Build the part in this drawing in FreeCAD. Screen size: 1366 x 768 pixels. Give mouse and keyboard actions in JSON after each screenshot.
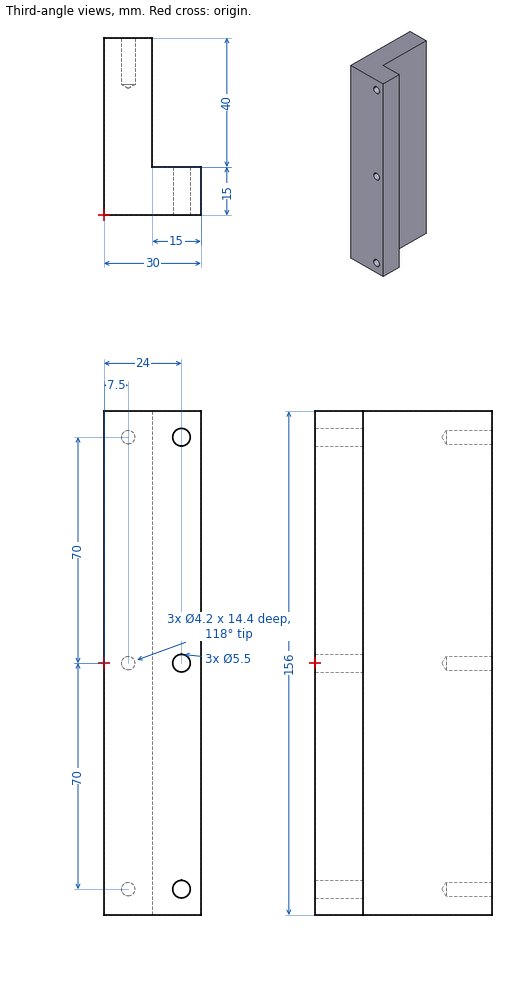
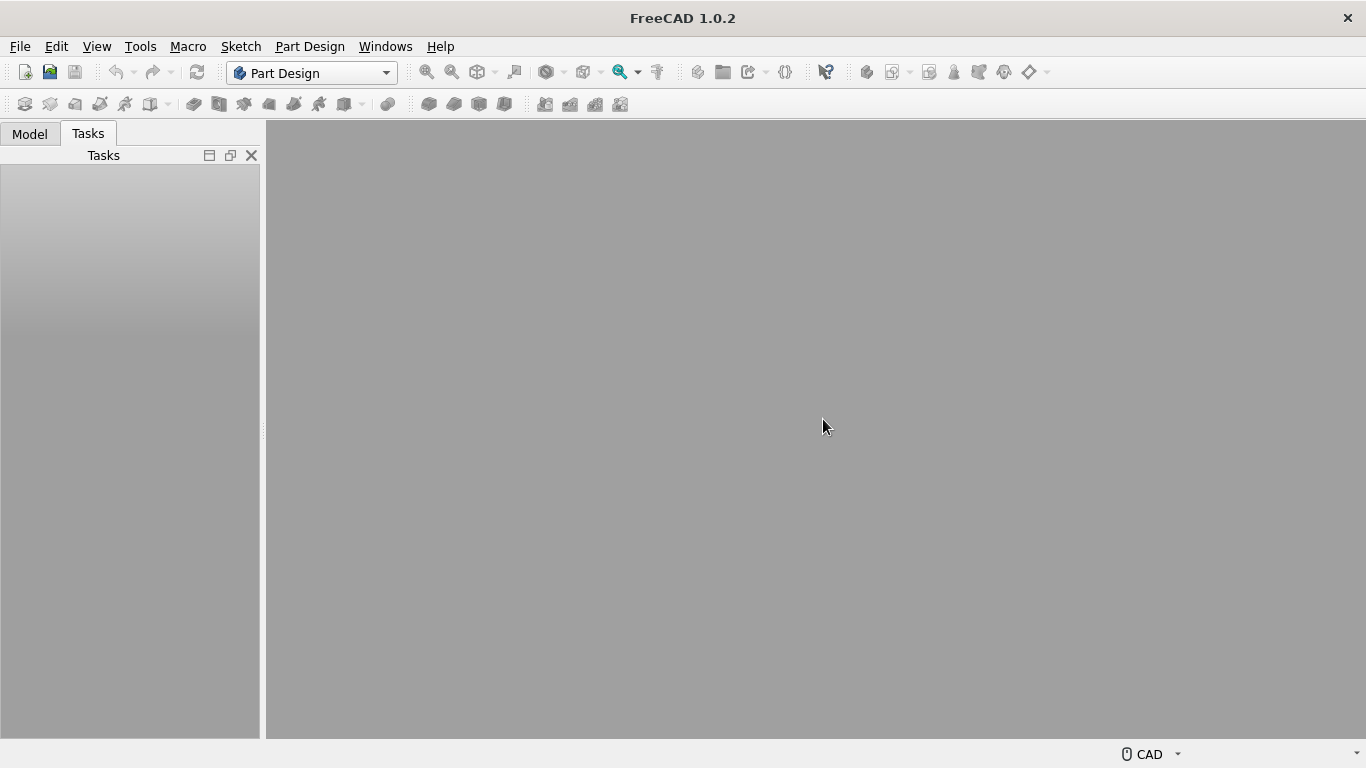
{"action": "key", "text": "ctrl+n"}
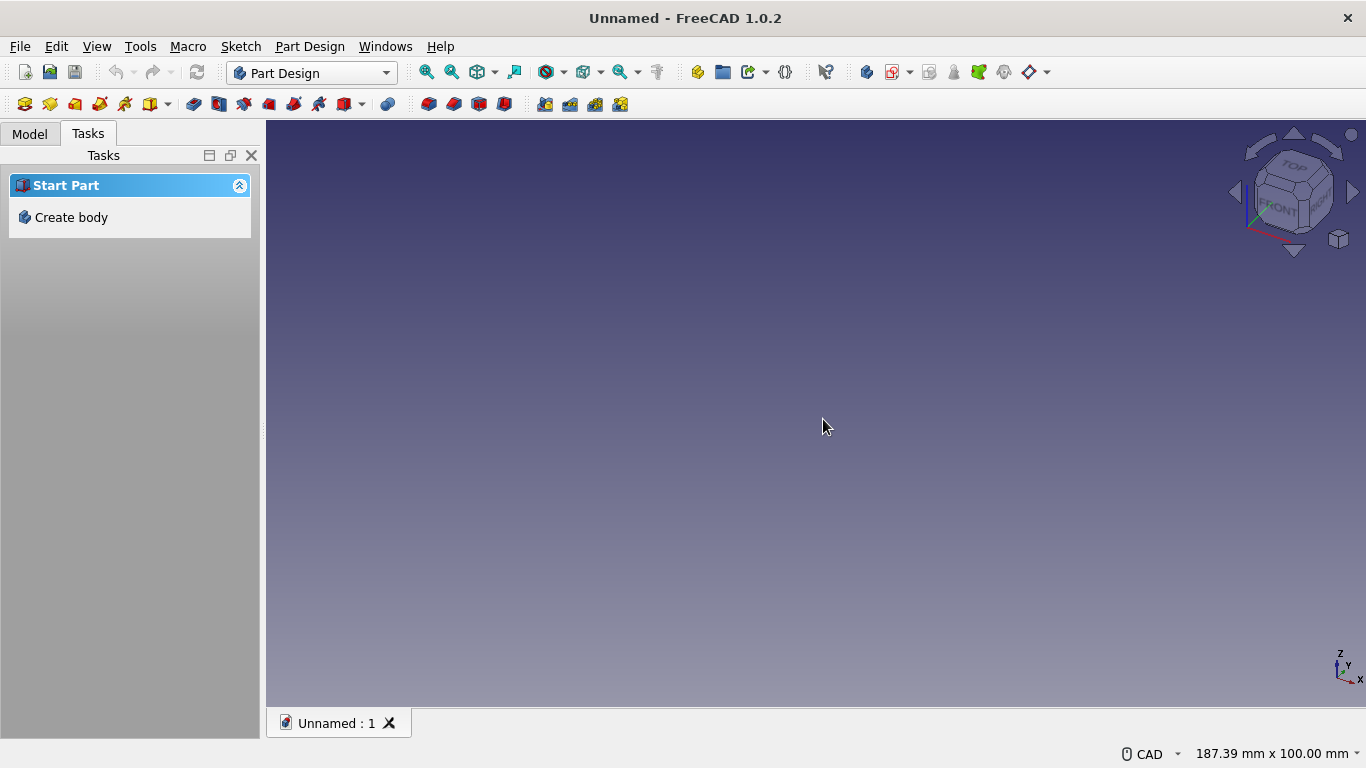
{"action": "left_click", "coordinate": [892, 72]}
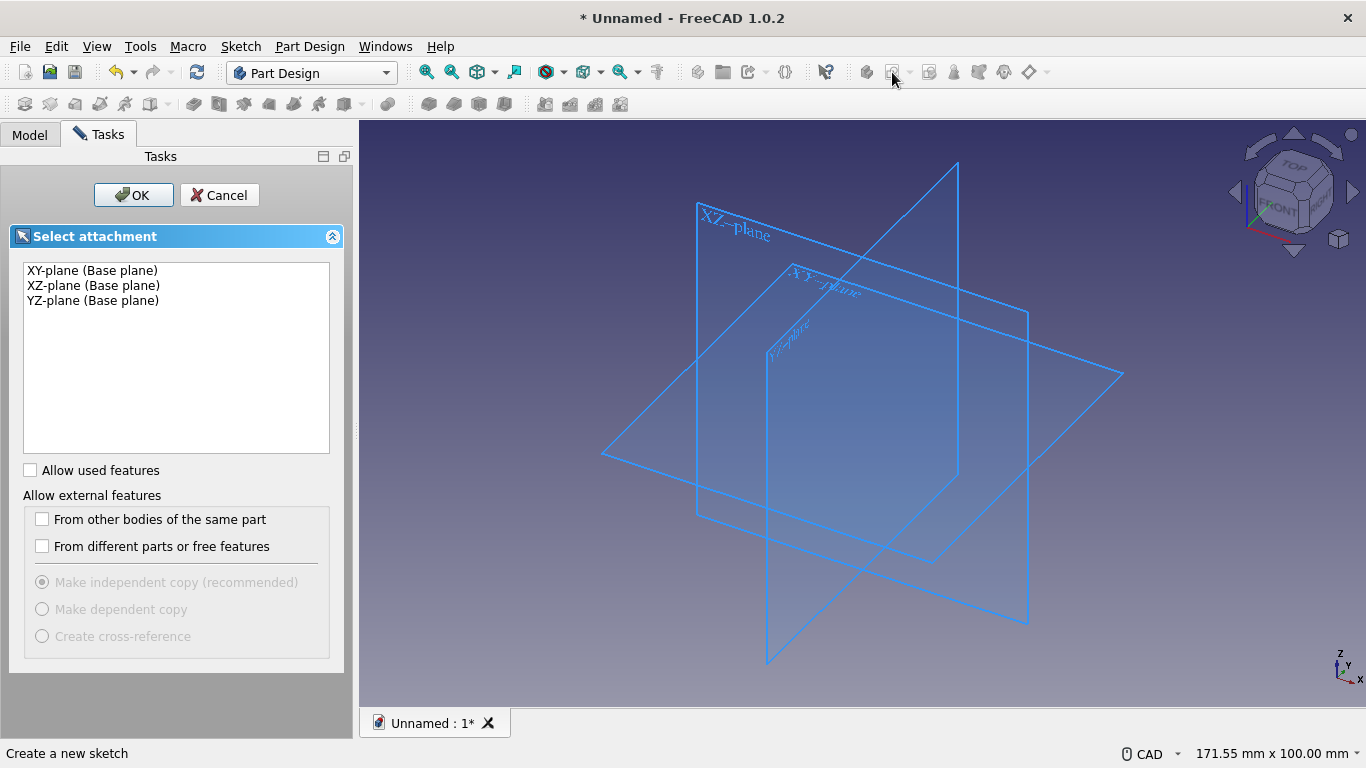
{"action": "left_click", "coordinate": [84, 270]}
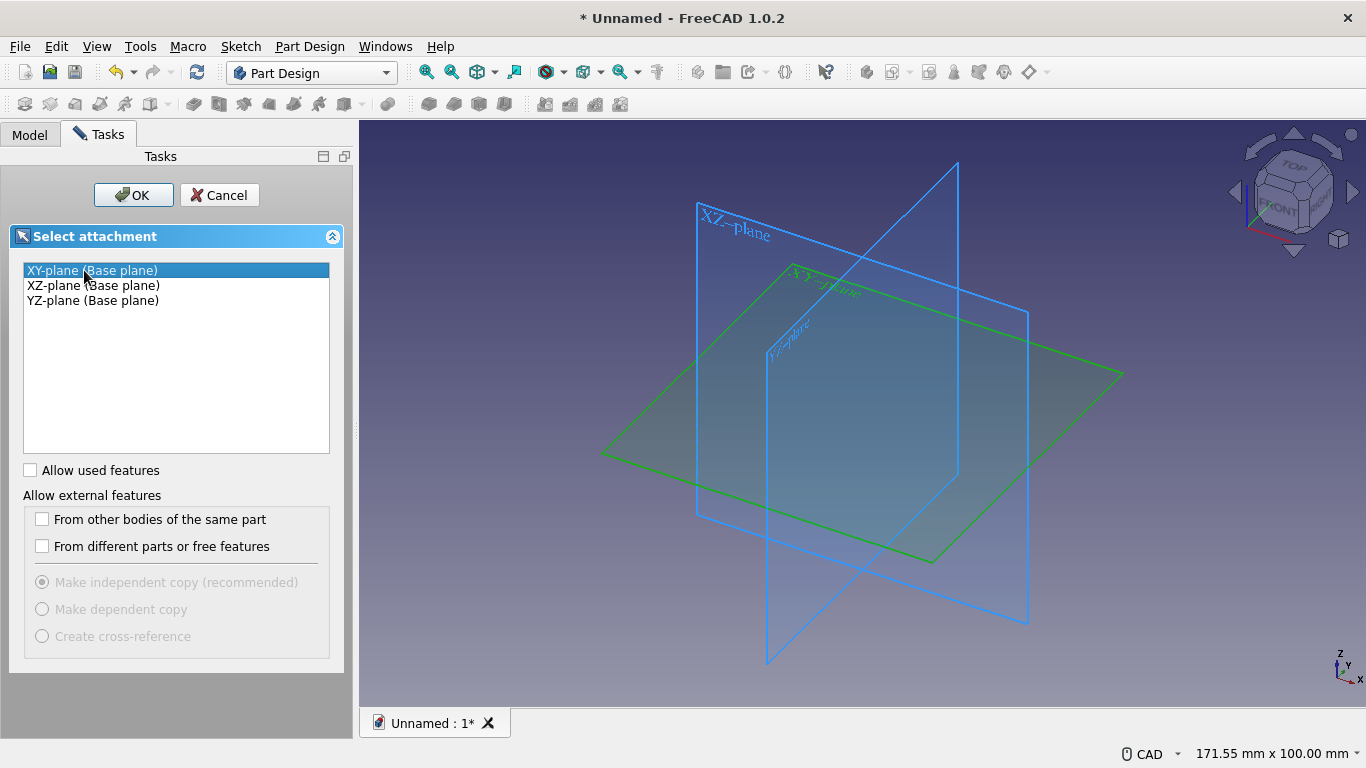
{"action": "left_click", "coordinate": [134, 195]}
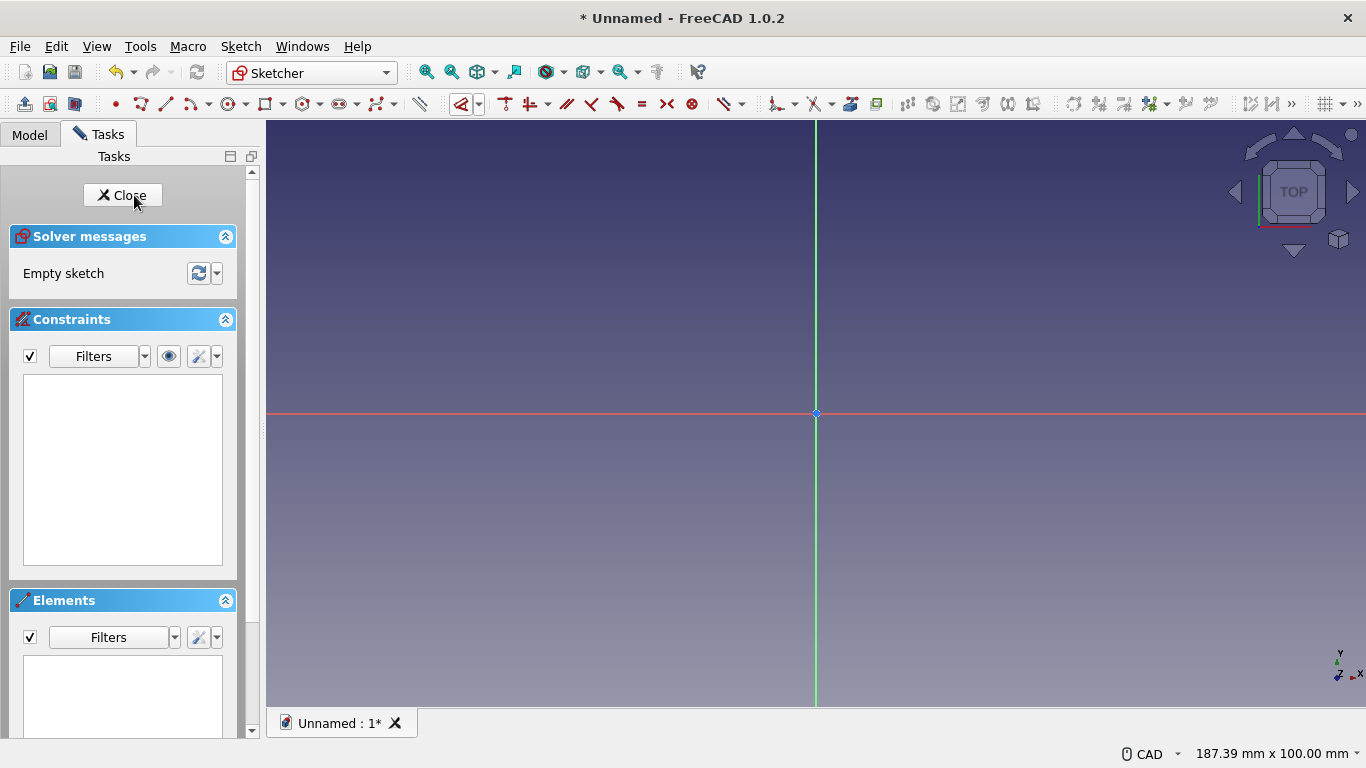
{"action": "scroll", "coordinate": [294, 679], "scroll_direction": "down", "scroll_amount": 1}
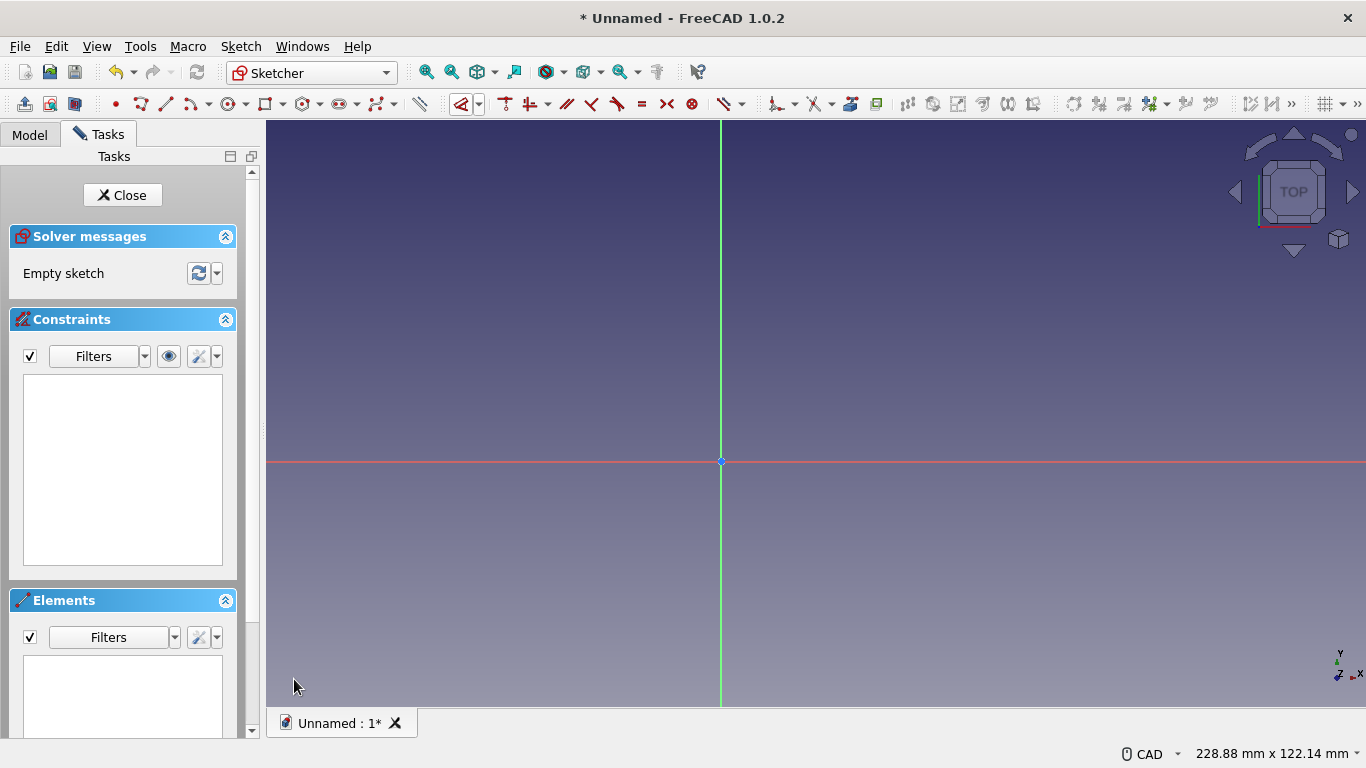
{"action": "scroll", "coordinate": [887, 159], "scroll_direction": "up", "scroll_amount": 2}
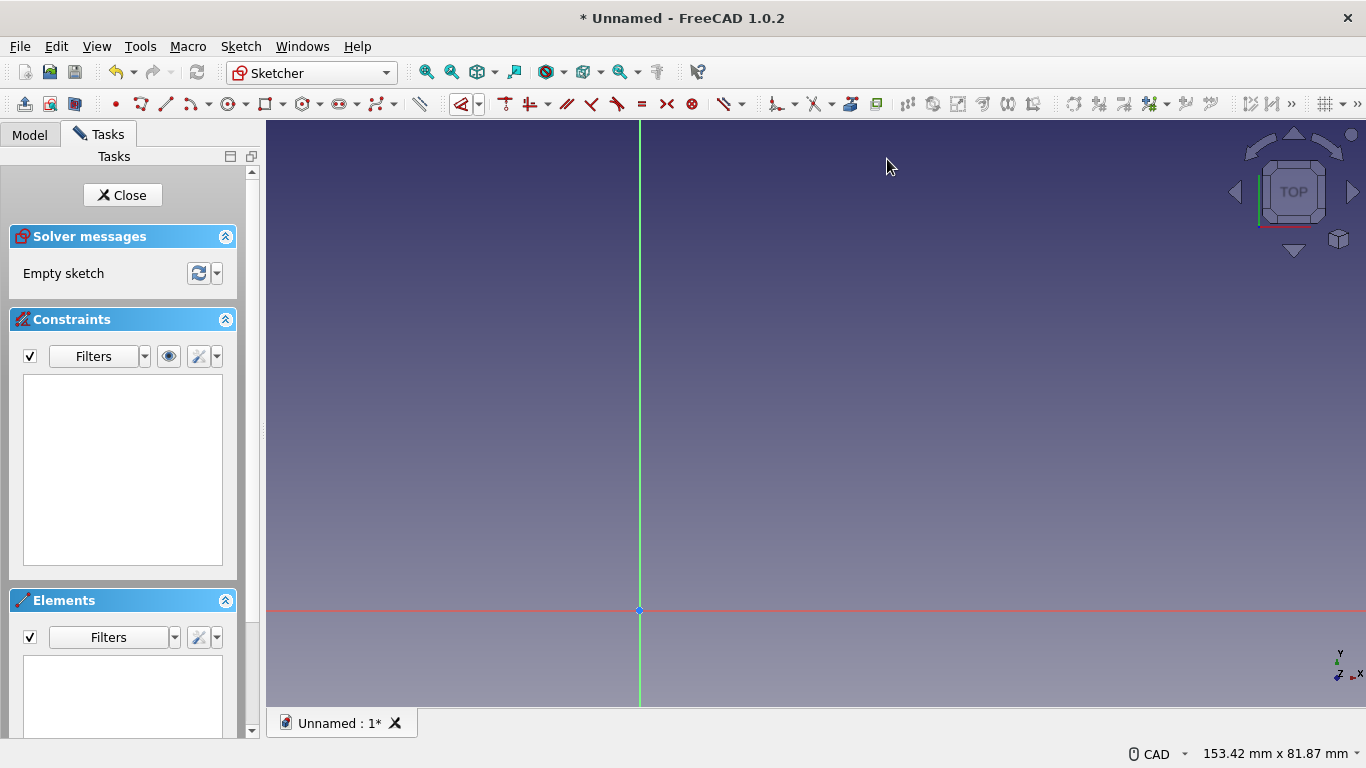
{"action": "key", "text": "g m"}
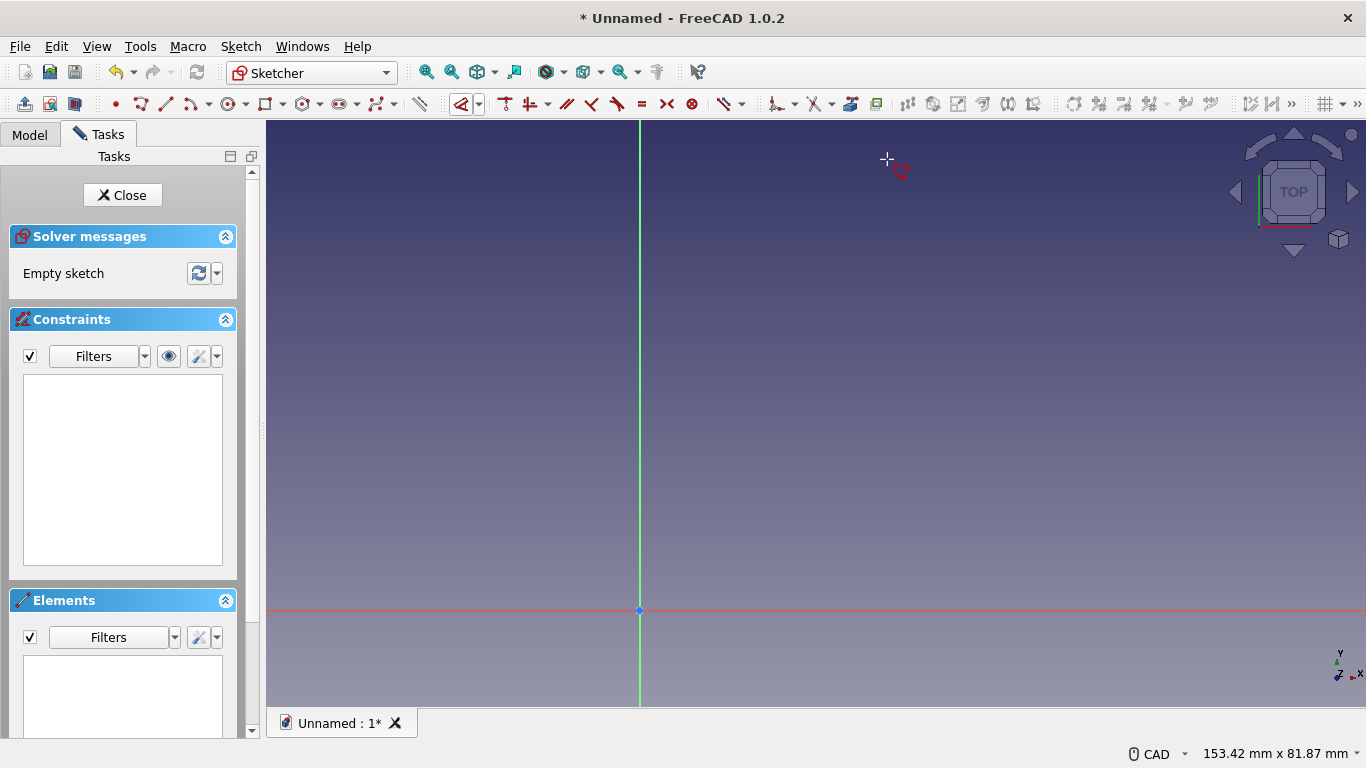
{"action": "left_click", "coordinate": [640, 611]}
{"action": "left_click", "coordinate": [855, 602]}
{"action": "left_click", "coordinate": [855, 503]}
{"action": "left_click", "coordinate": [747, 503]}
{"action": "left_click", "coordinate": [747, 216]}
{"action": "left_click", "coordinate": [649, 216]}
{"action": "left_click", "coordinate": [640, 611]}
{"action": "key", "text": "Escape"}
{"action": "key", "text": "Escape"}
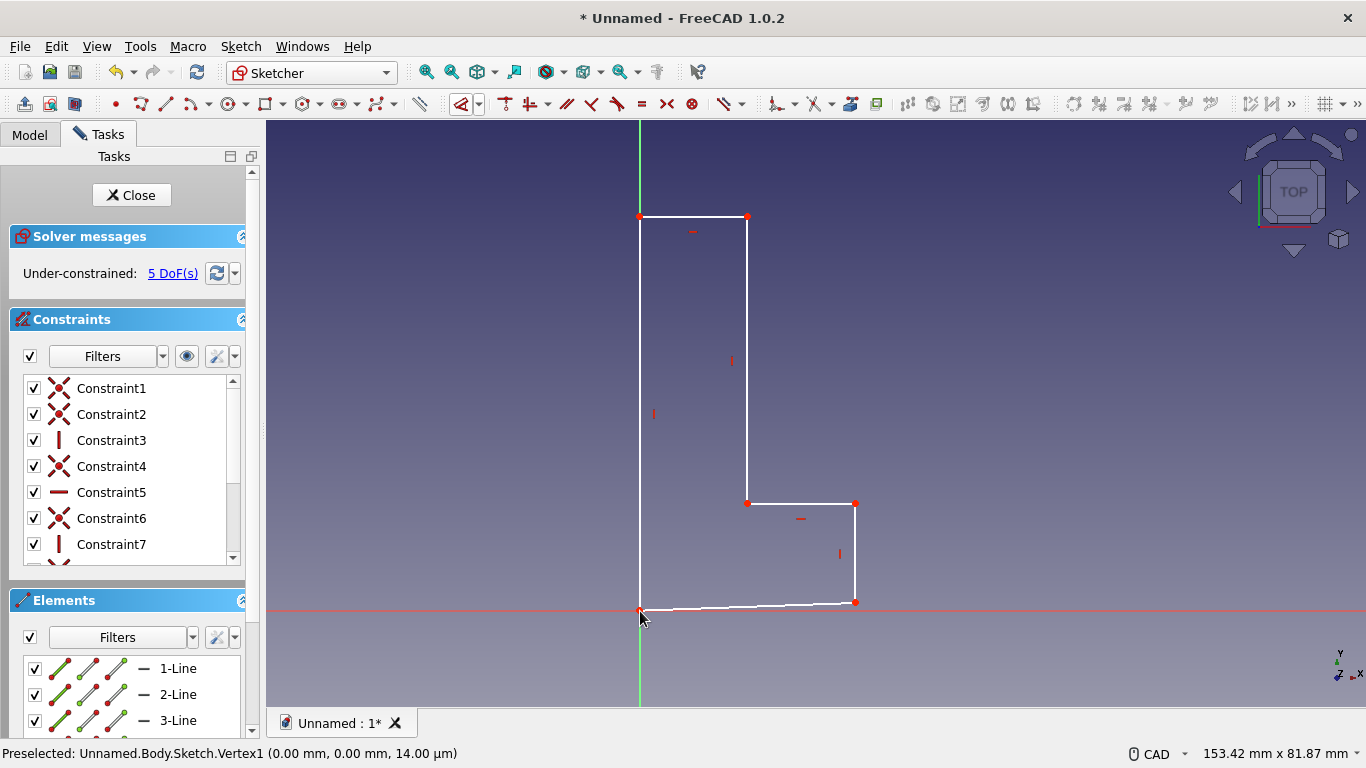
{"action": "left_click", "coordinate": [704, 608]}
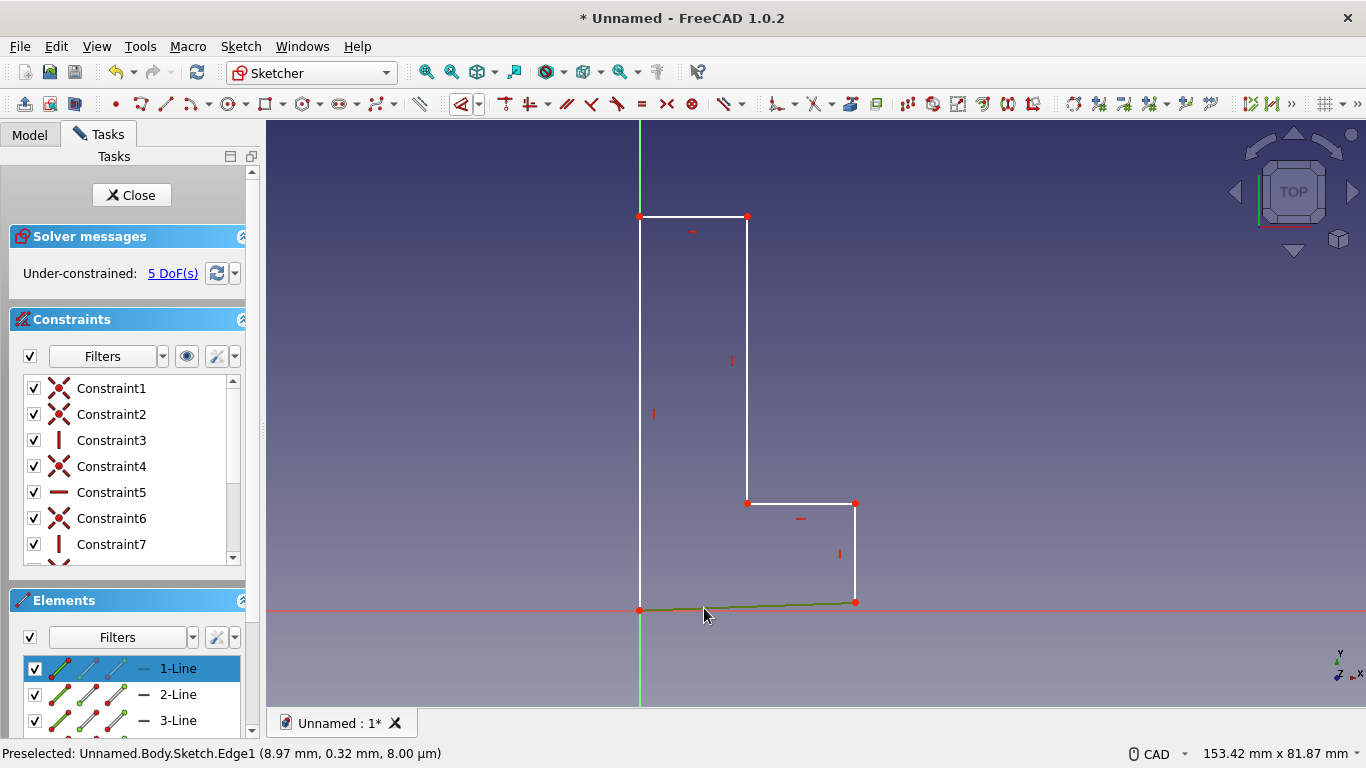
{"action": "key", "text": "h"}